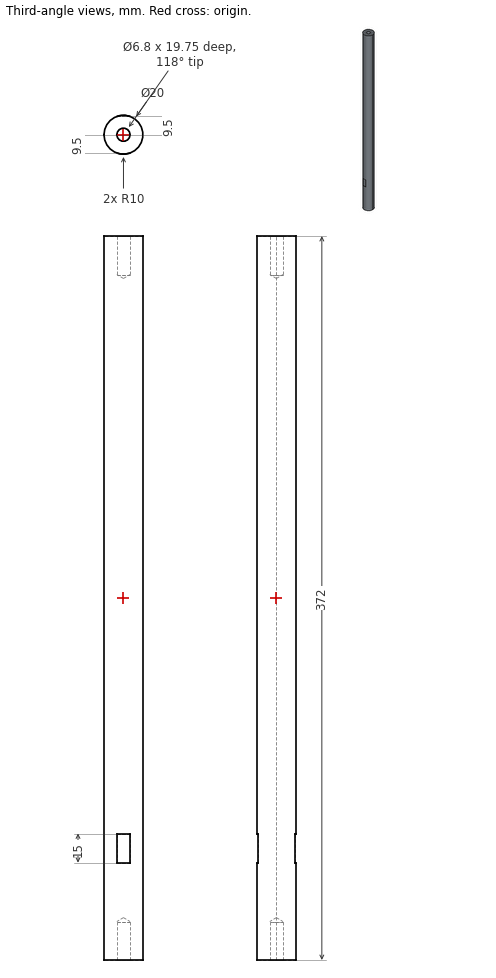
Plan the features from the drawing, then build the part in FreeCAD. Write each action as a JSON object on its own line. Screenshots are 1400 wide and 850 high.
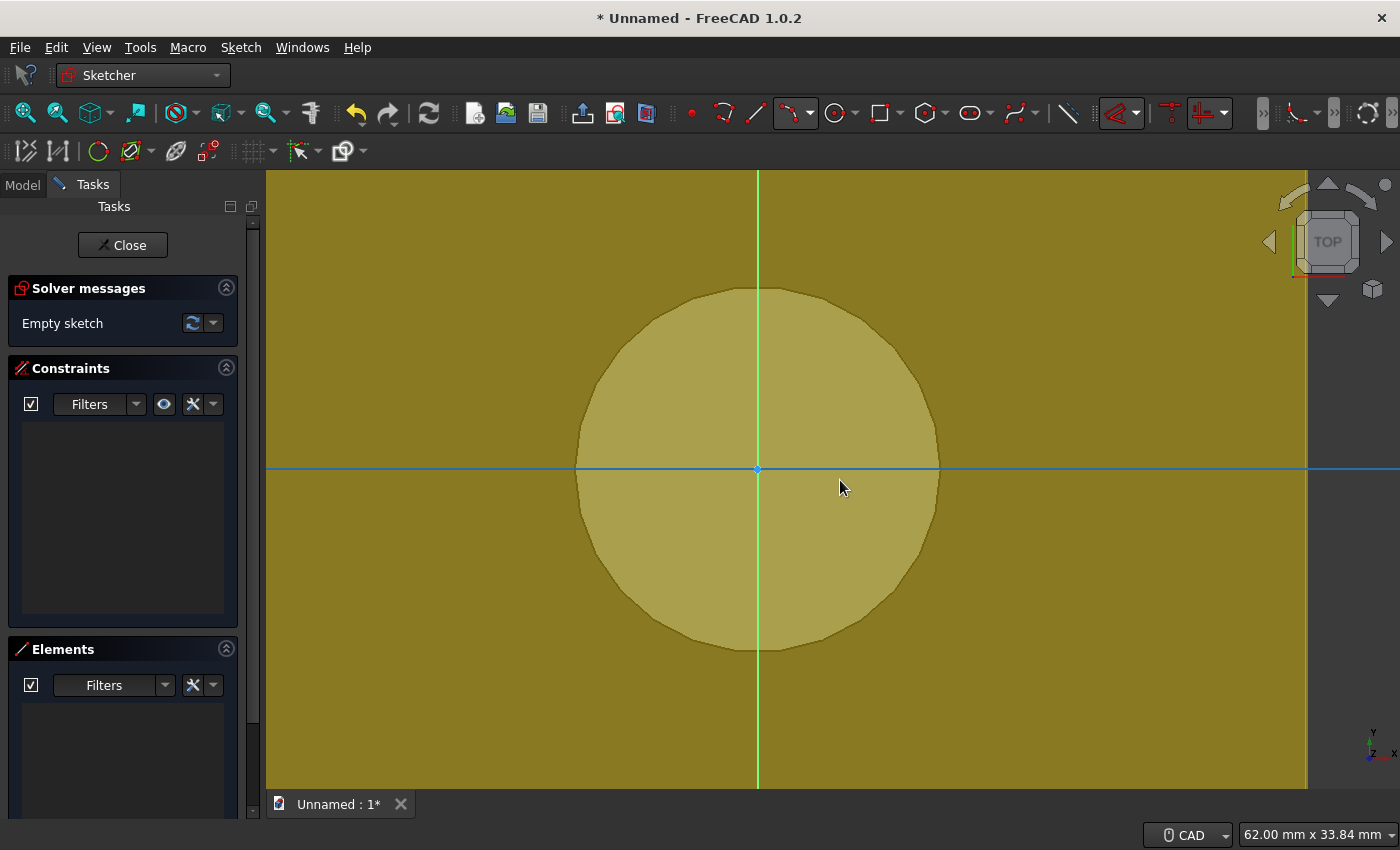
{"action": "key", "text": "g l"}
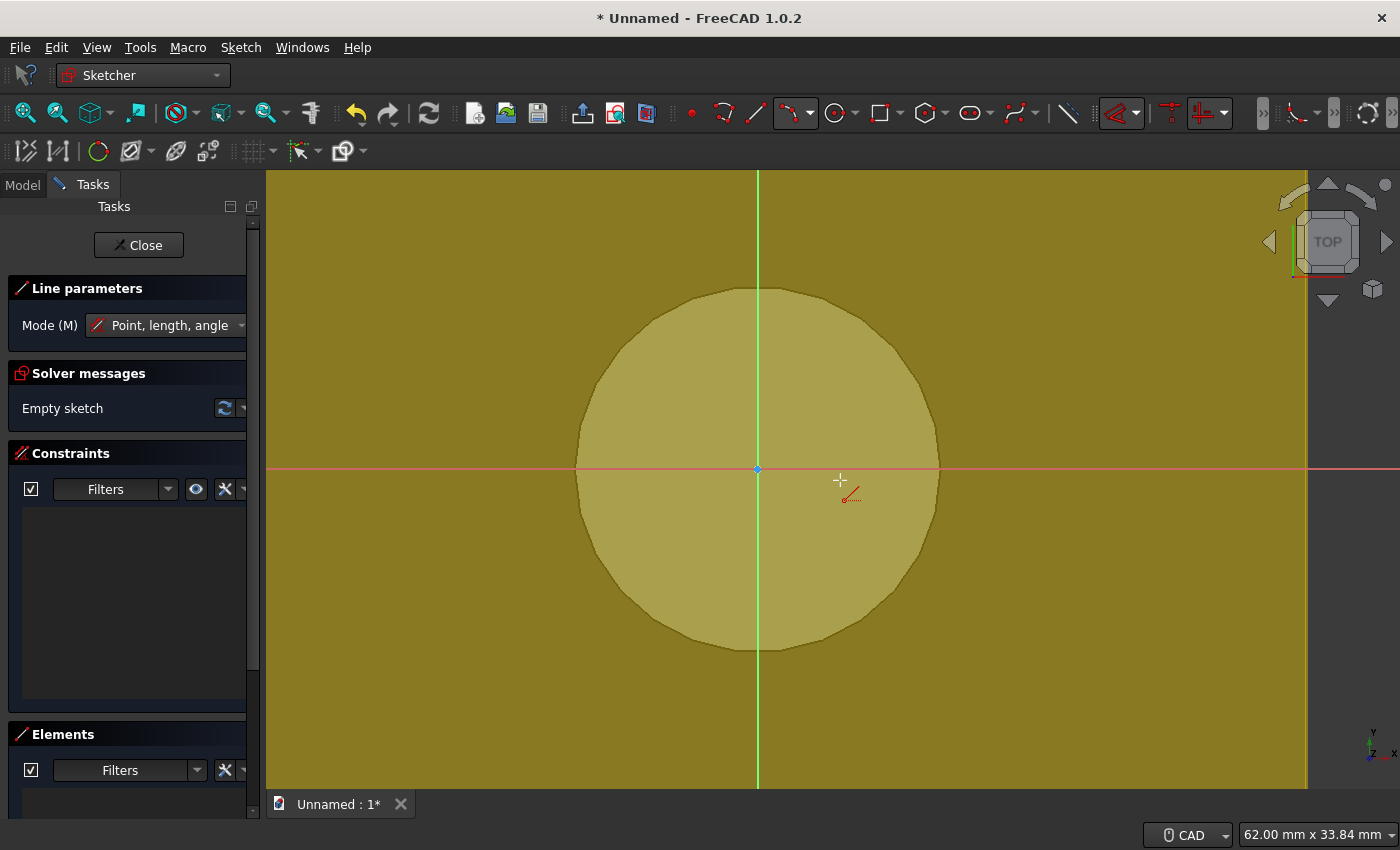
{"action": "left_click", "coordinate": [701, 643]}
{"action": "left_click", "coordinate": [815, 643]}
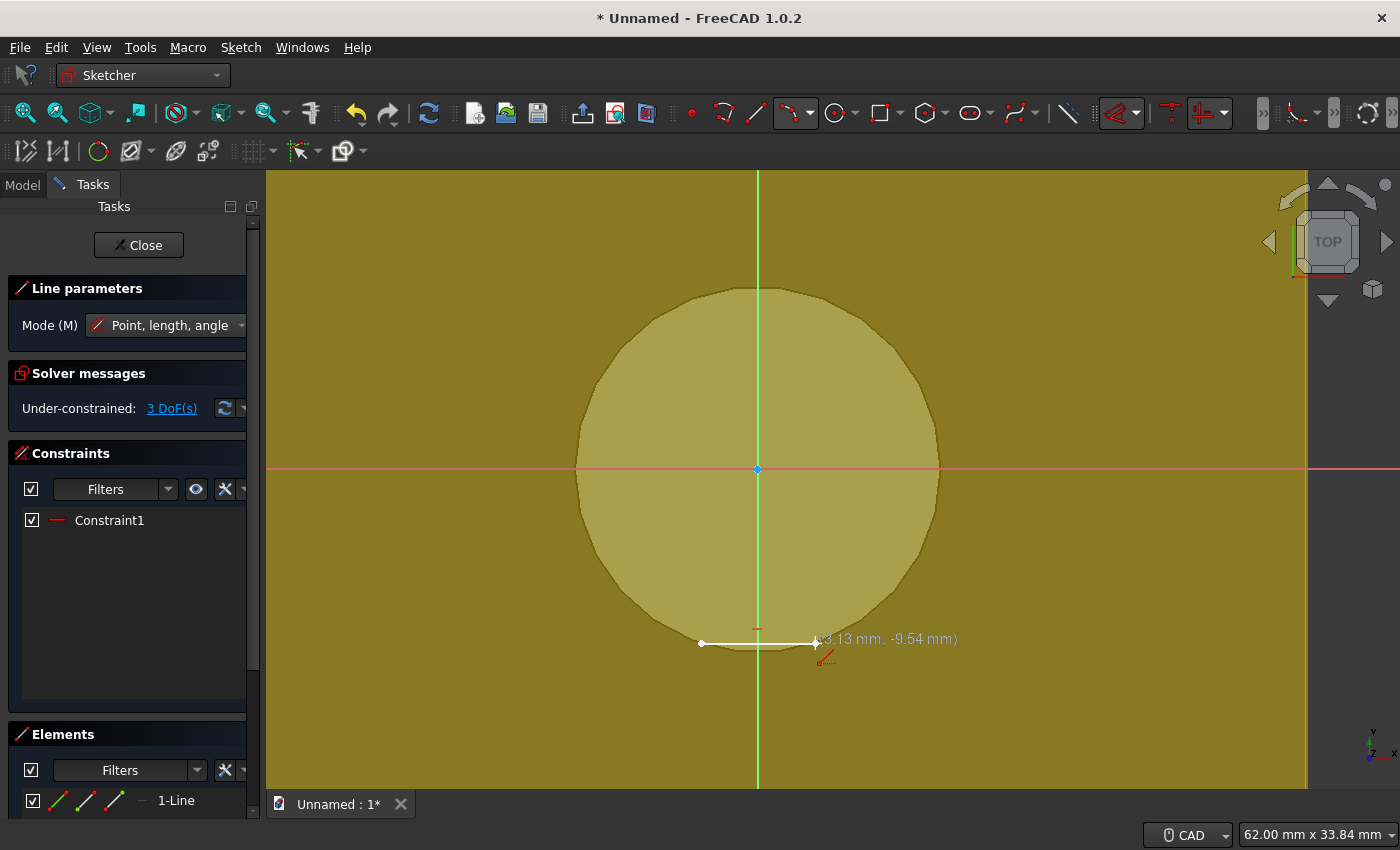
{"action": "left_click", "coordinate": [790, 114]}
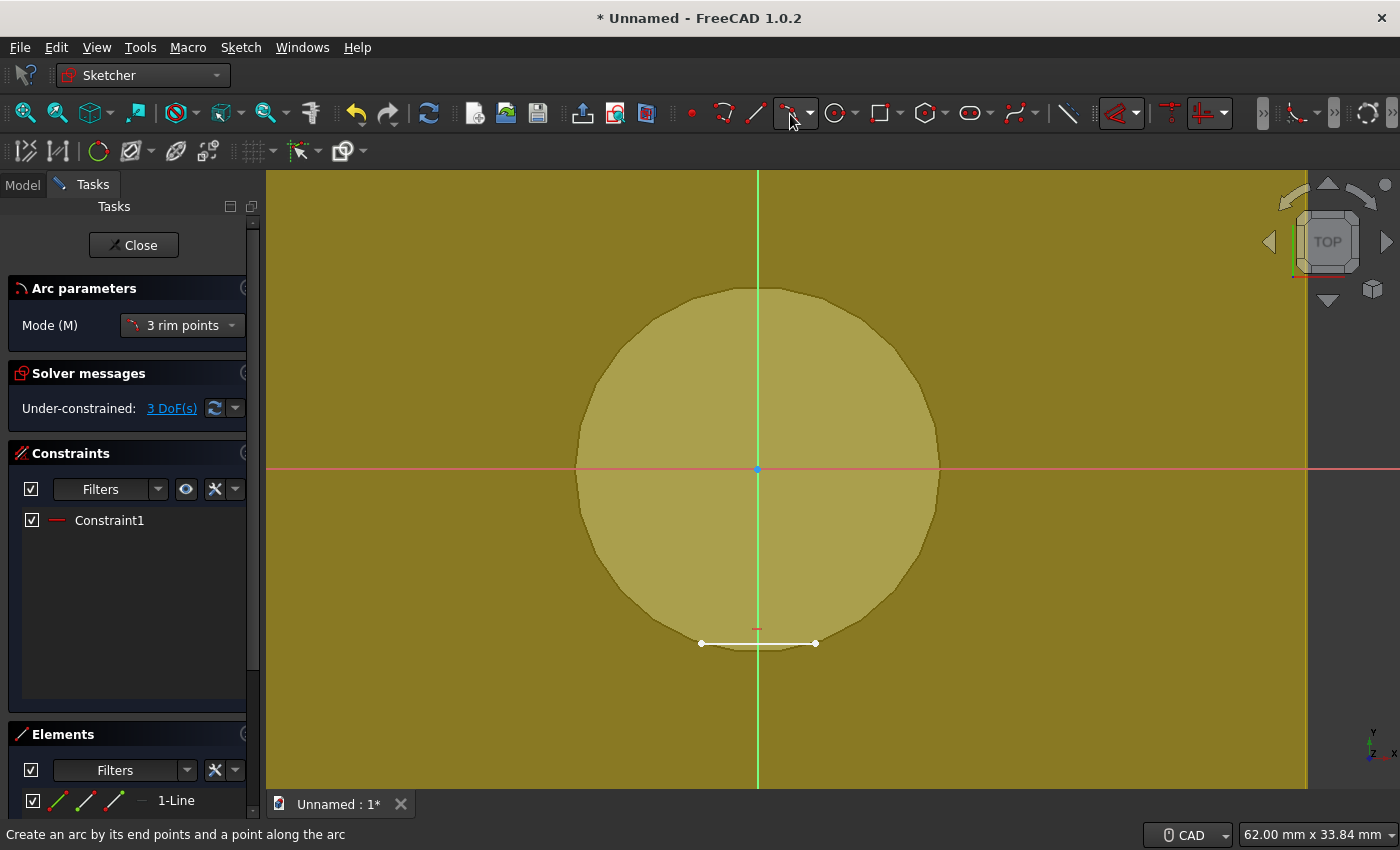
{"action": "left_click", "coordinate": [815, 644]}
{"action": "left_click", "coordinate": [701, 644]}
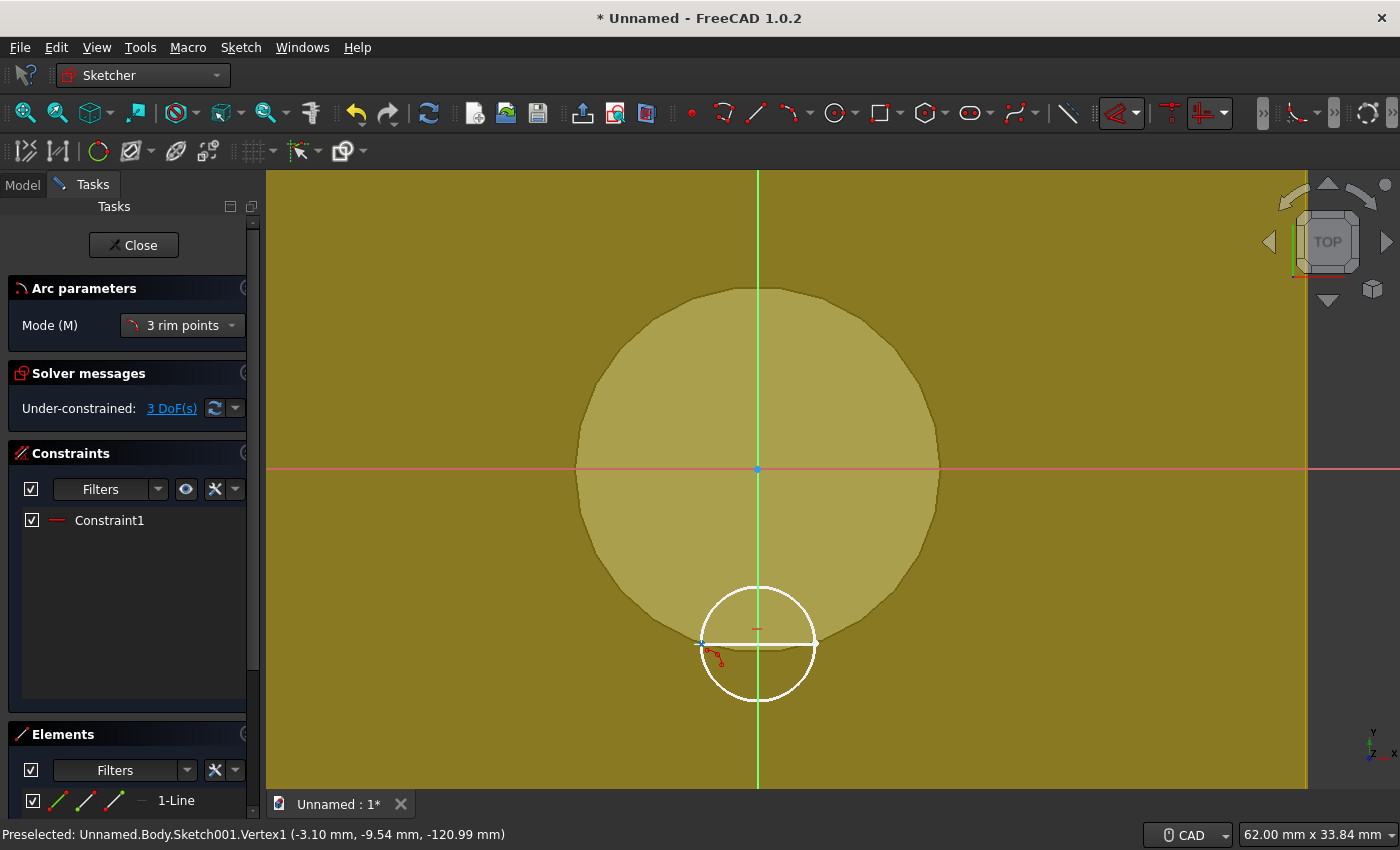
{"action": "scroll", "coordinate": [746, 652], "scroll_direction": "up", "scroll_amount": 3}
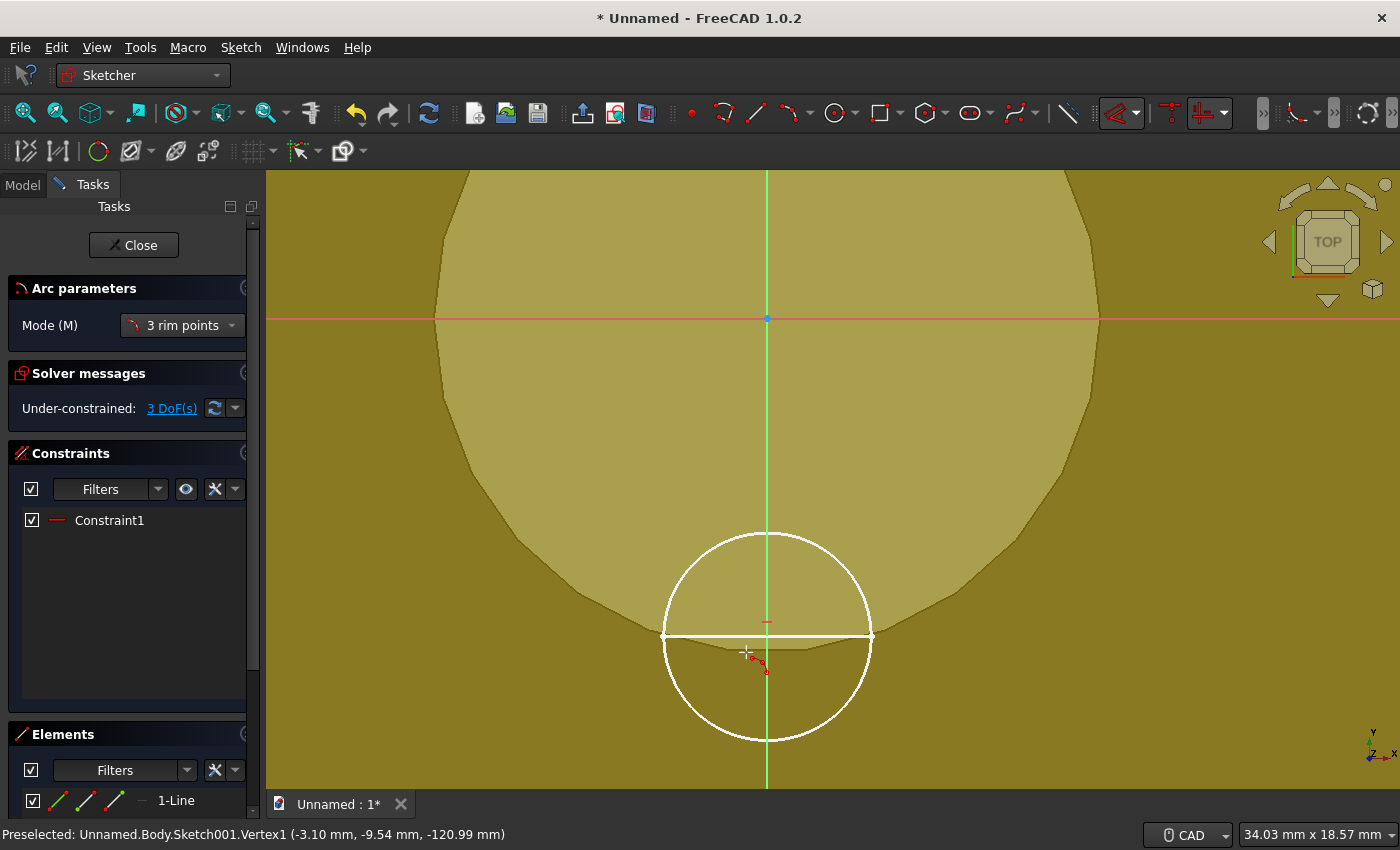
{"action": "left_click", "coordinate": [746, 651]}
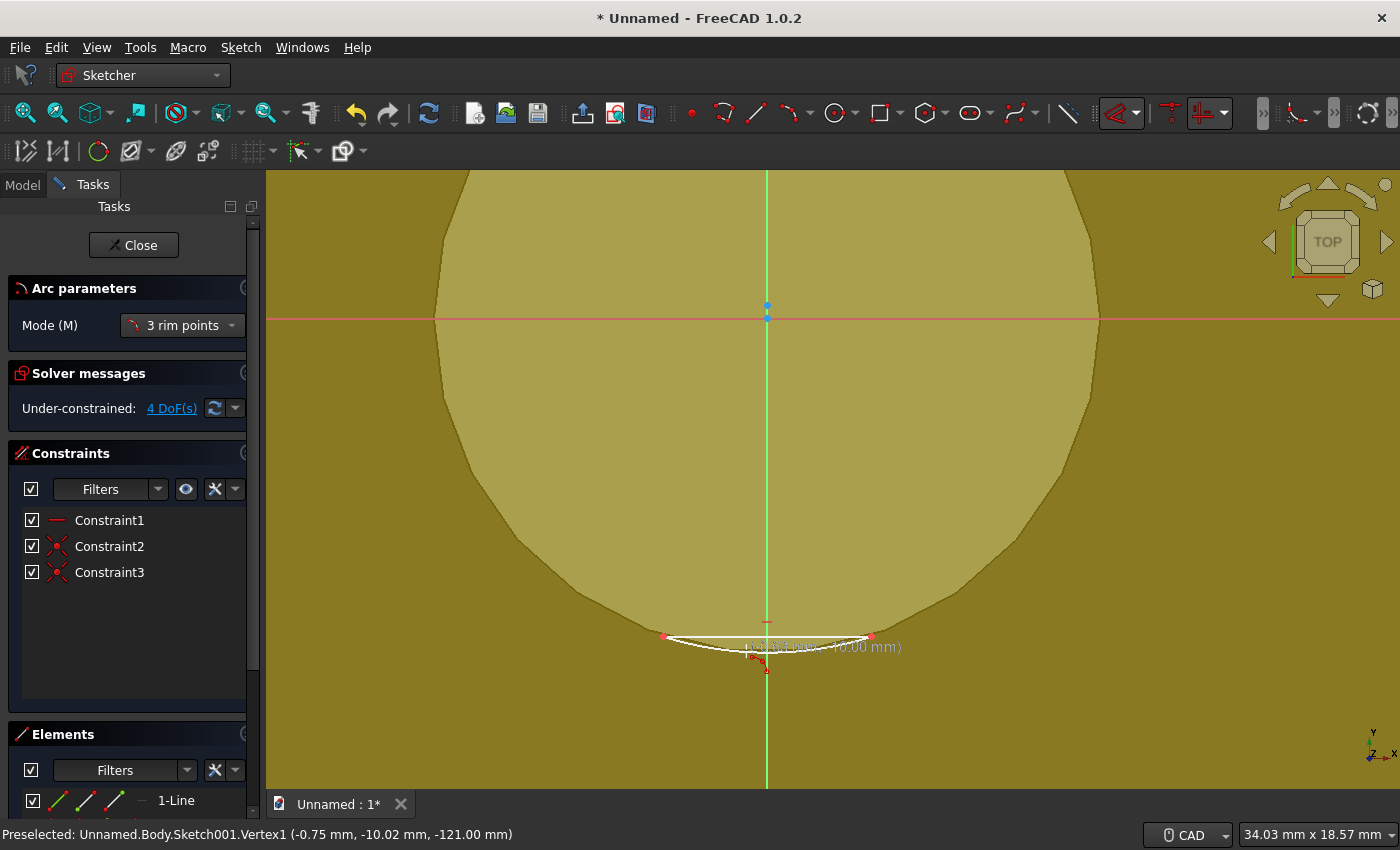
{"action": "left_click", "coordinate": [756, 114]}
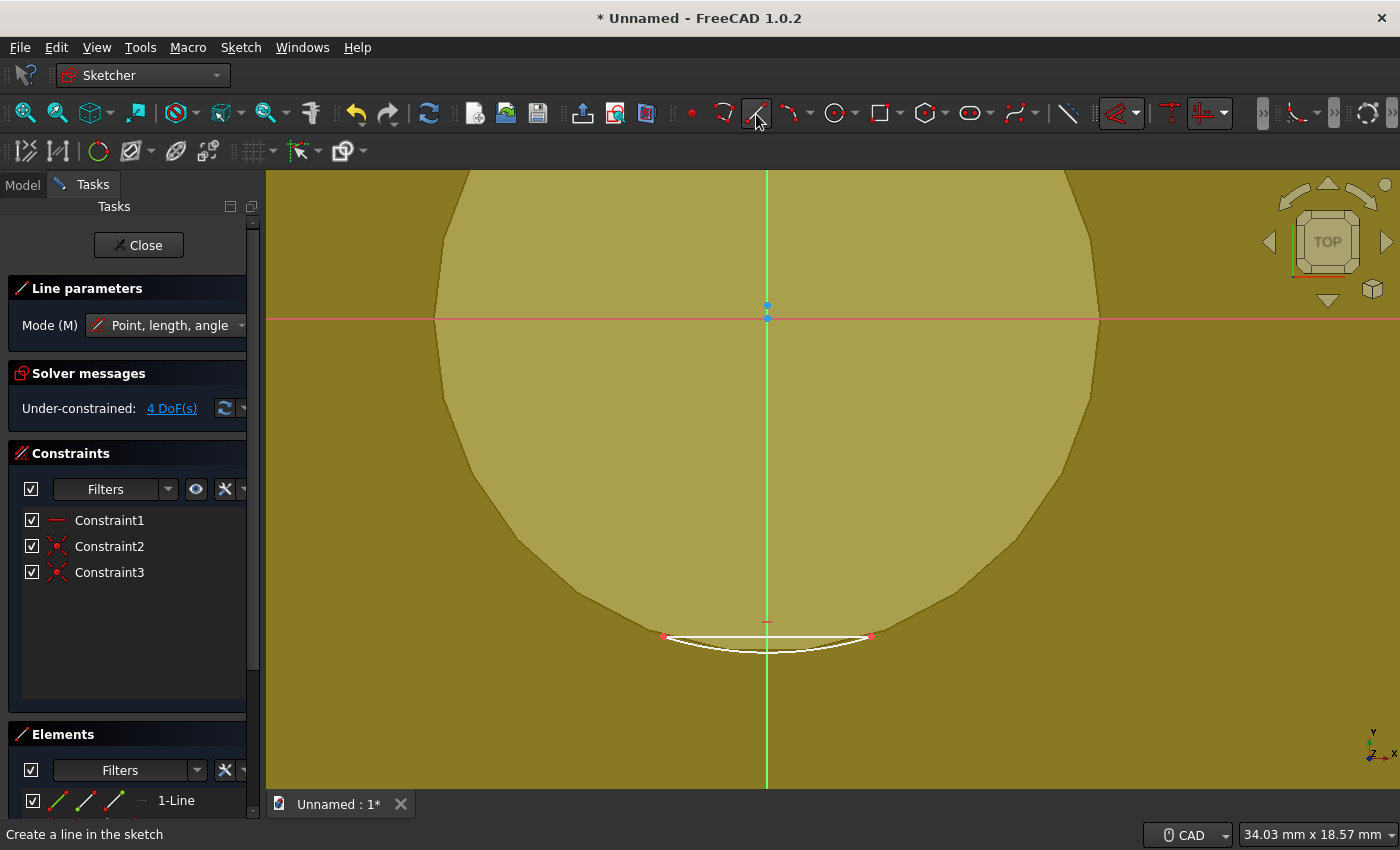
{"action": "scroll", "coordinate": [761, 675], "scroll_direction": "down", "scroll_amount": 3}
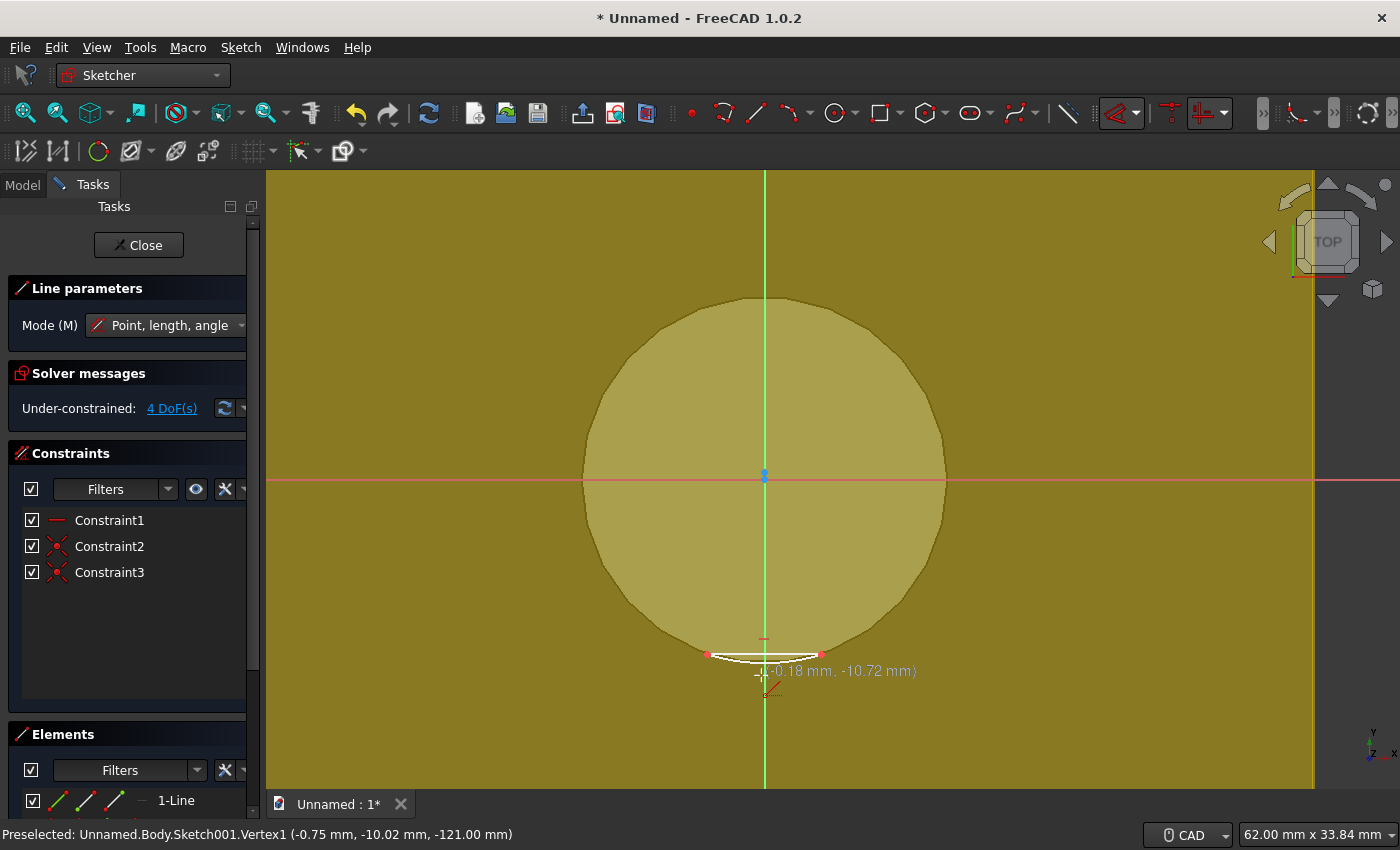
{"action": "left_click", "coordinate": [822, 306]}
{"action": "left_click", "coordinate": [707, 306]}